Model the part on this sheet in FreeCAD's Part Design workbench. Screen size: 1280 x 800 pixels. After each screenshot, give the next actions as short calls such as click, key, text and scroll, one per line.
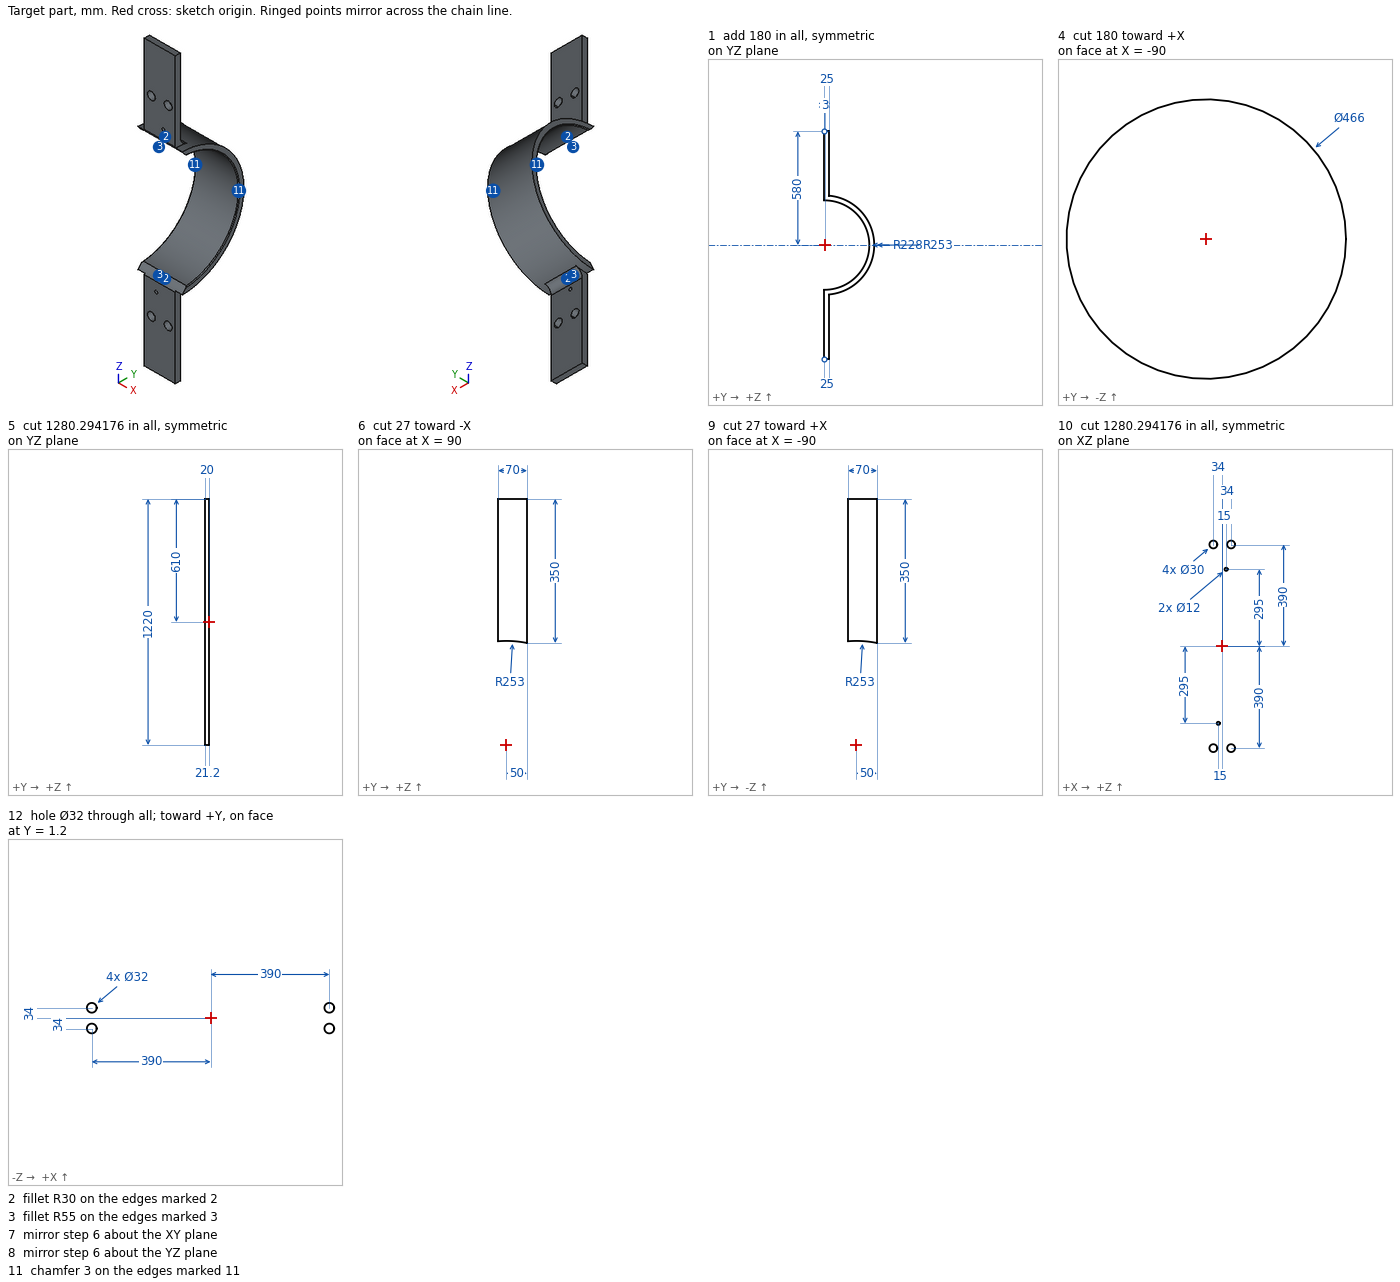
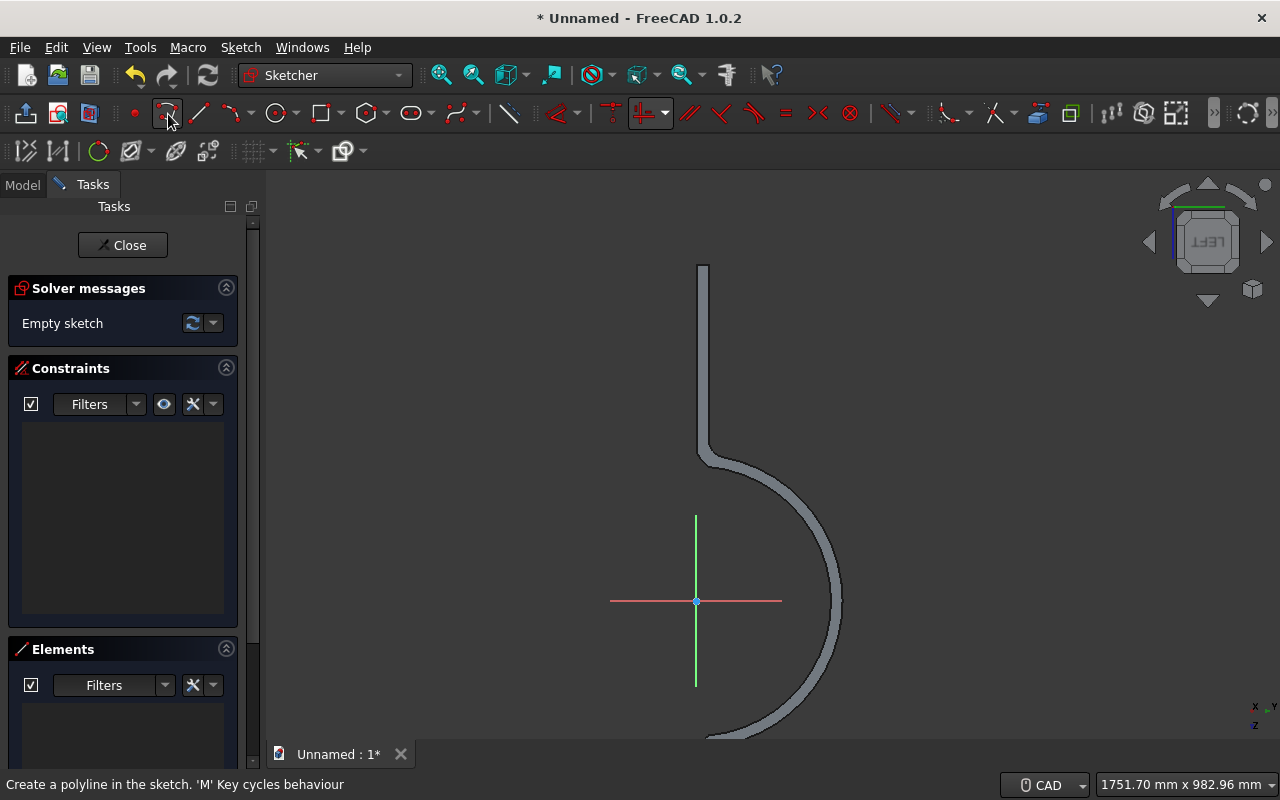
click(725, 458)
click(725, 255)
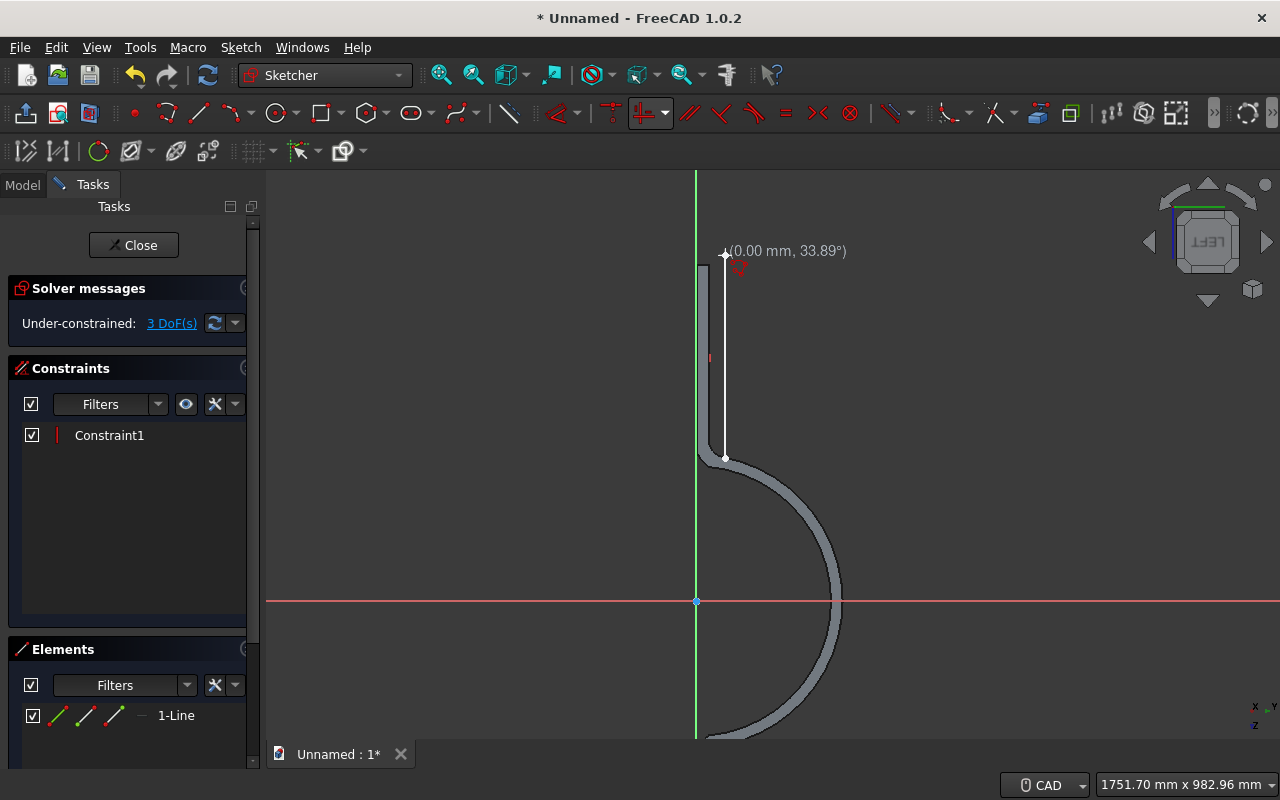
scroll(685, 255, up, 2)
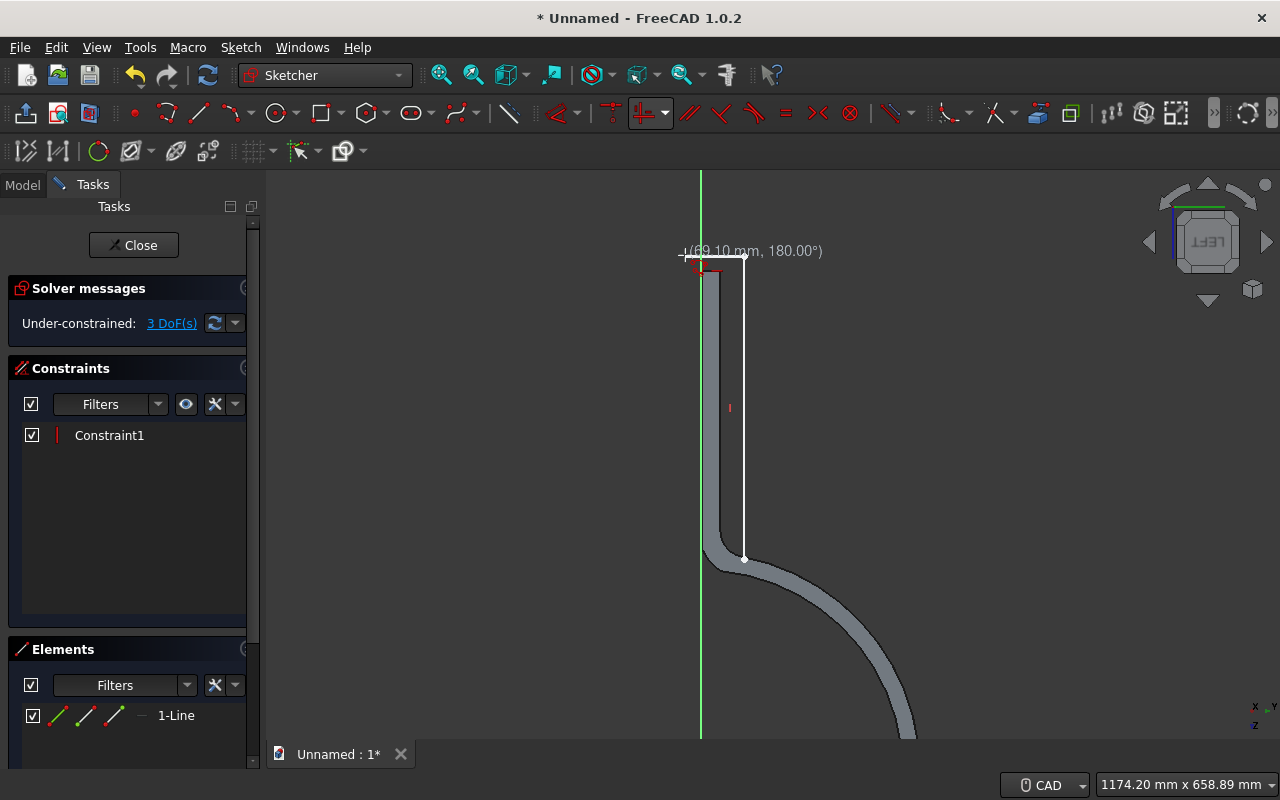
click(684, 255)
click(684, 554)
right_click(684, 554)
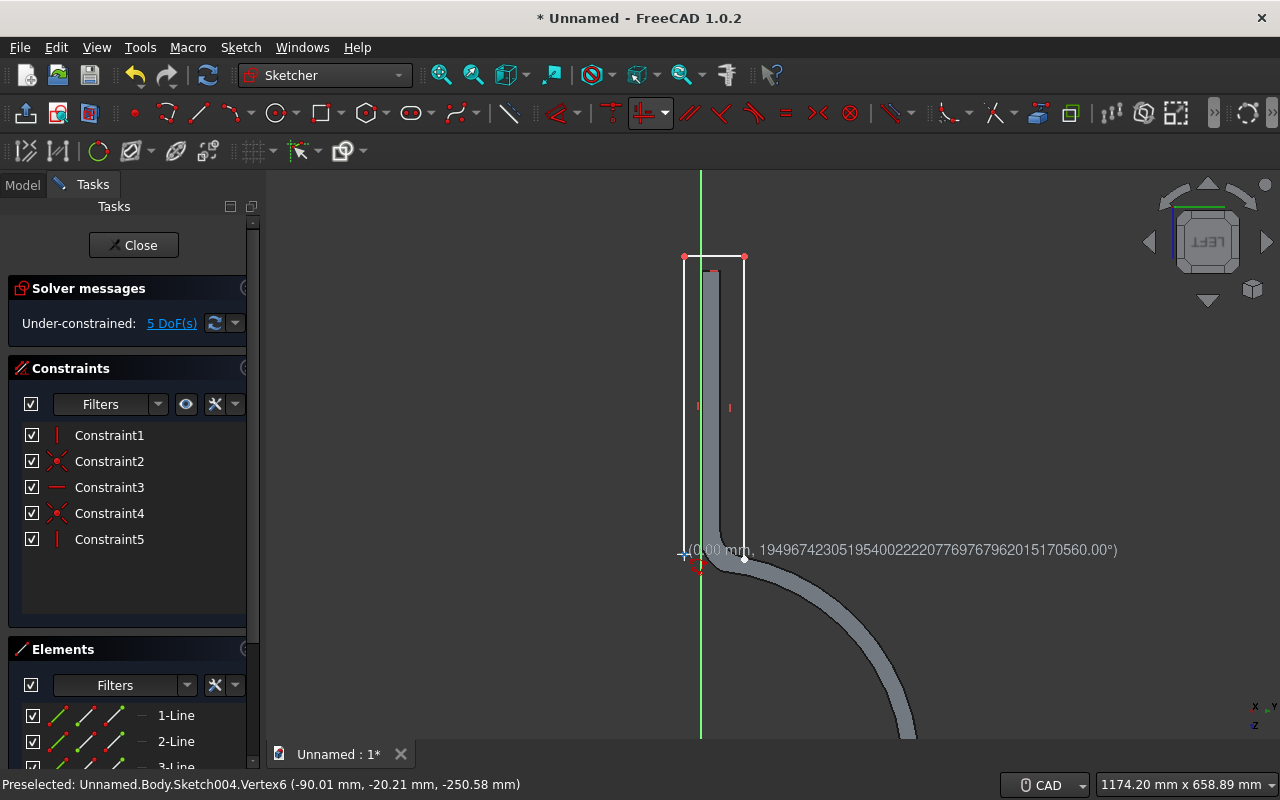
click(232, 114)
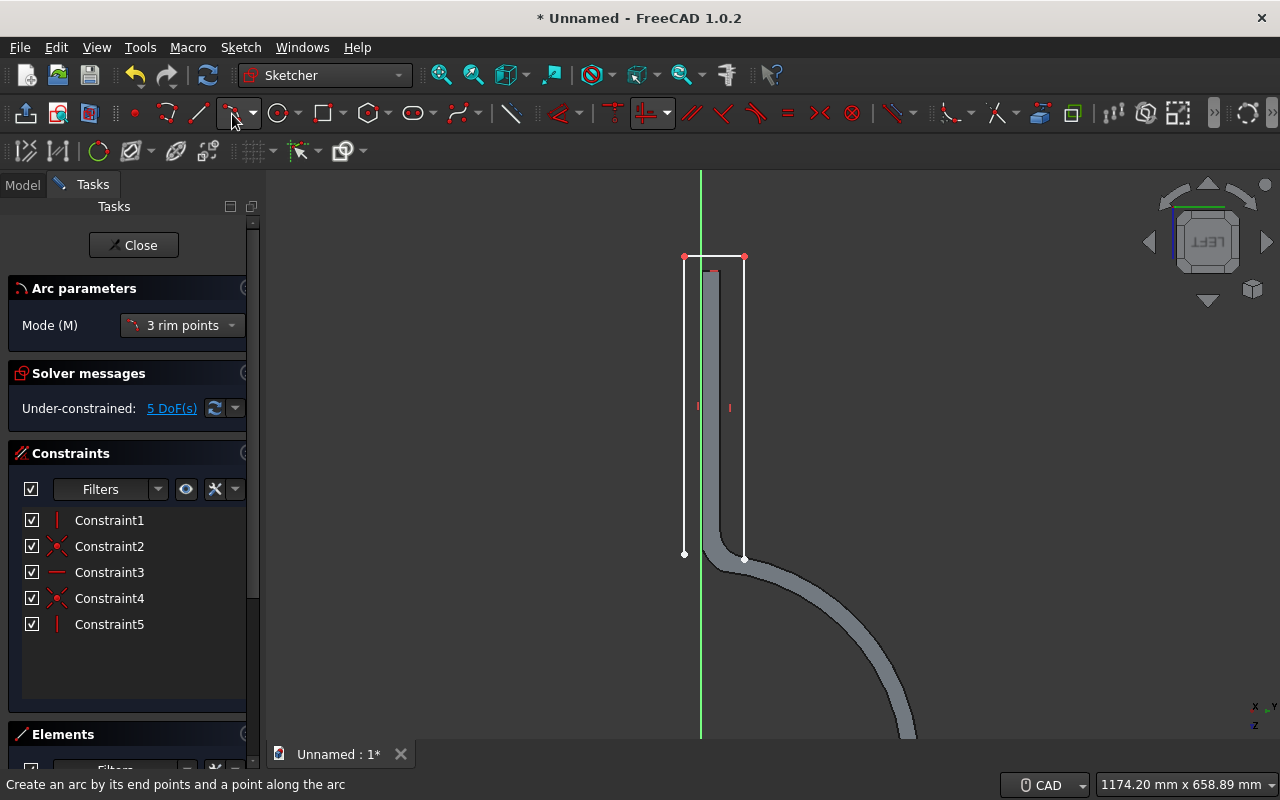
click(684, 555)
click(744, 559)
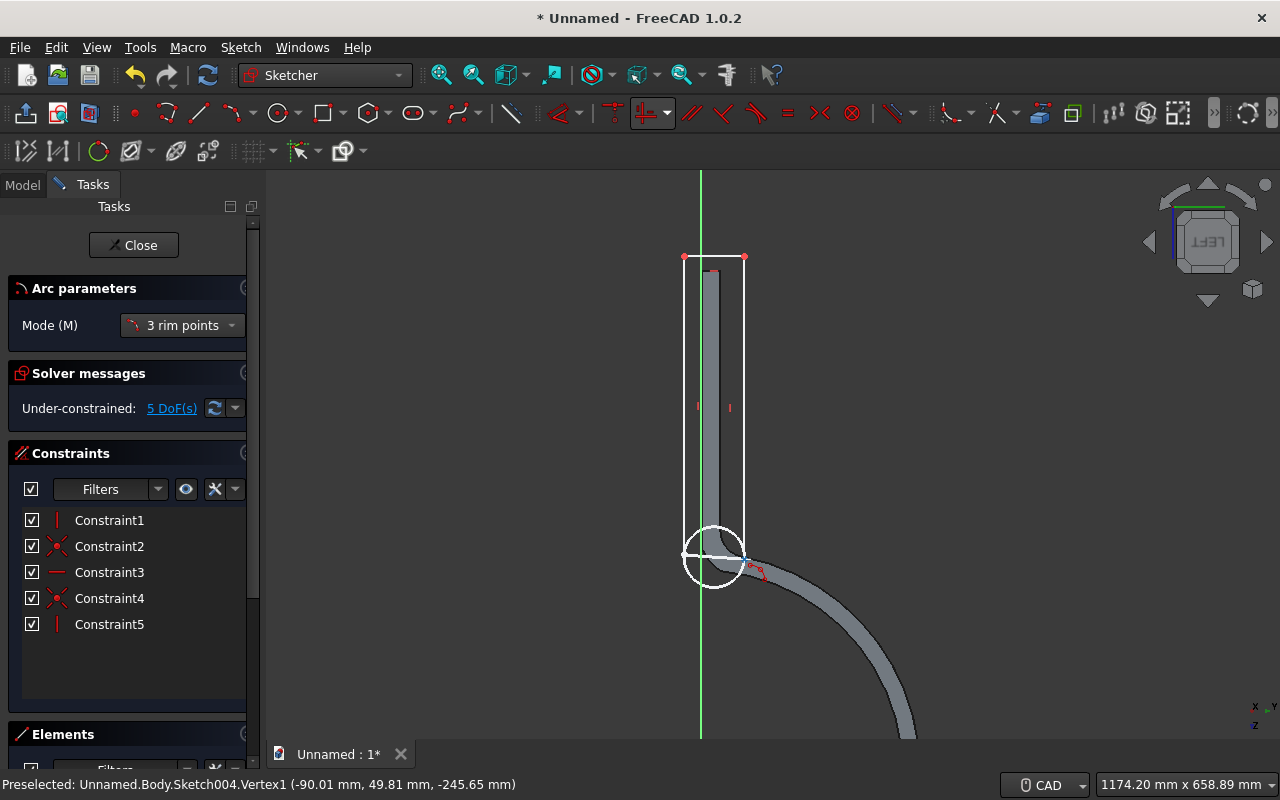
scroll(715, 553, up, 11)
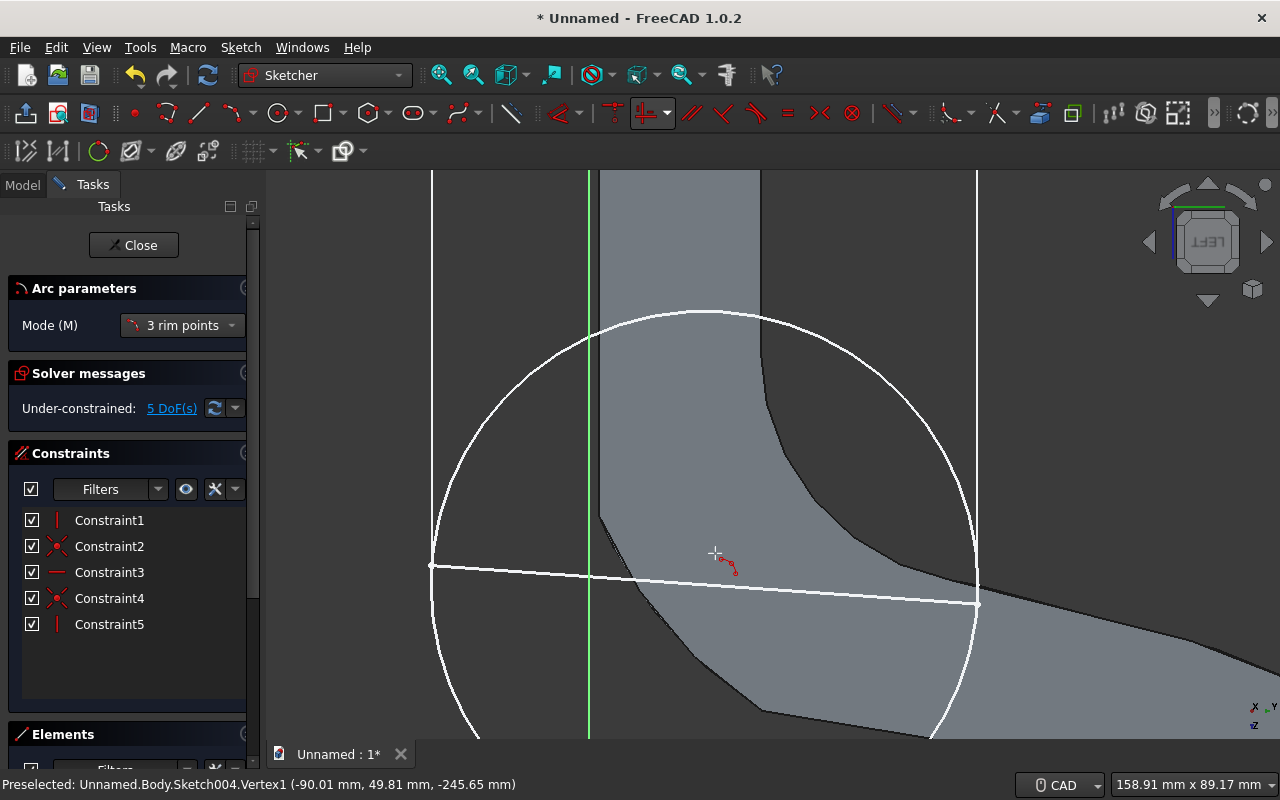
click(707, 550)
key(Escape)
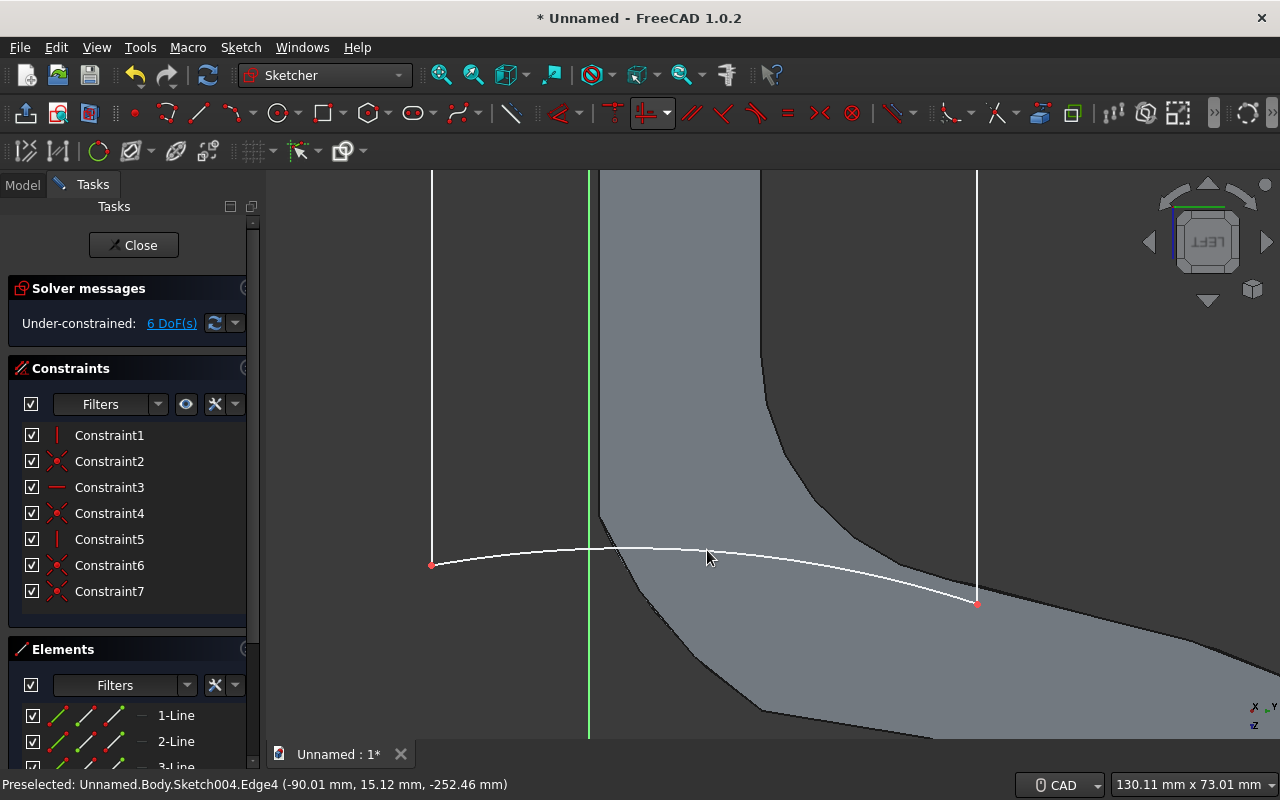
scroll(704, 476, down, 13)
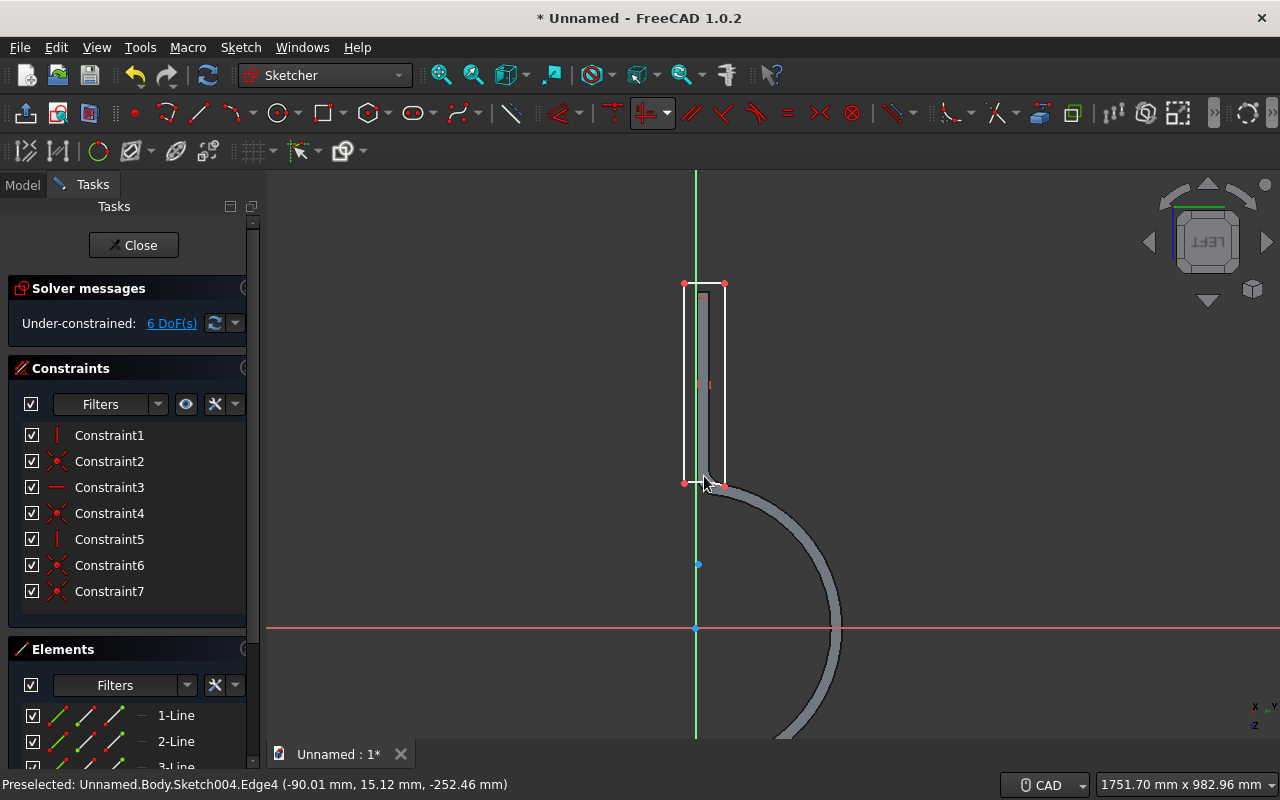
drag(686, 555, 709, 638)